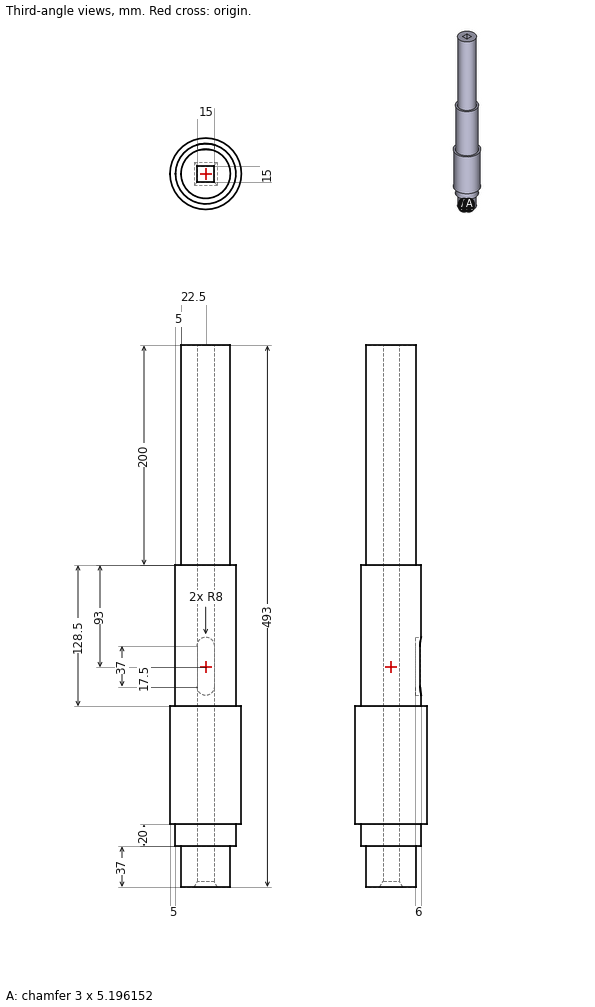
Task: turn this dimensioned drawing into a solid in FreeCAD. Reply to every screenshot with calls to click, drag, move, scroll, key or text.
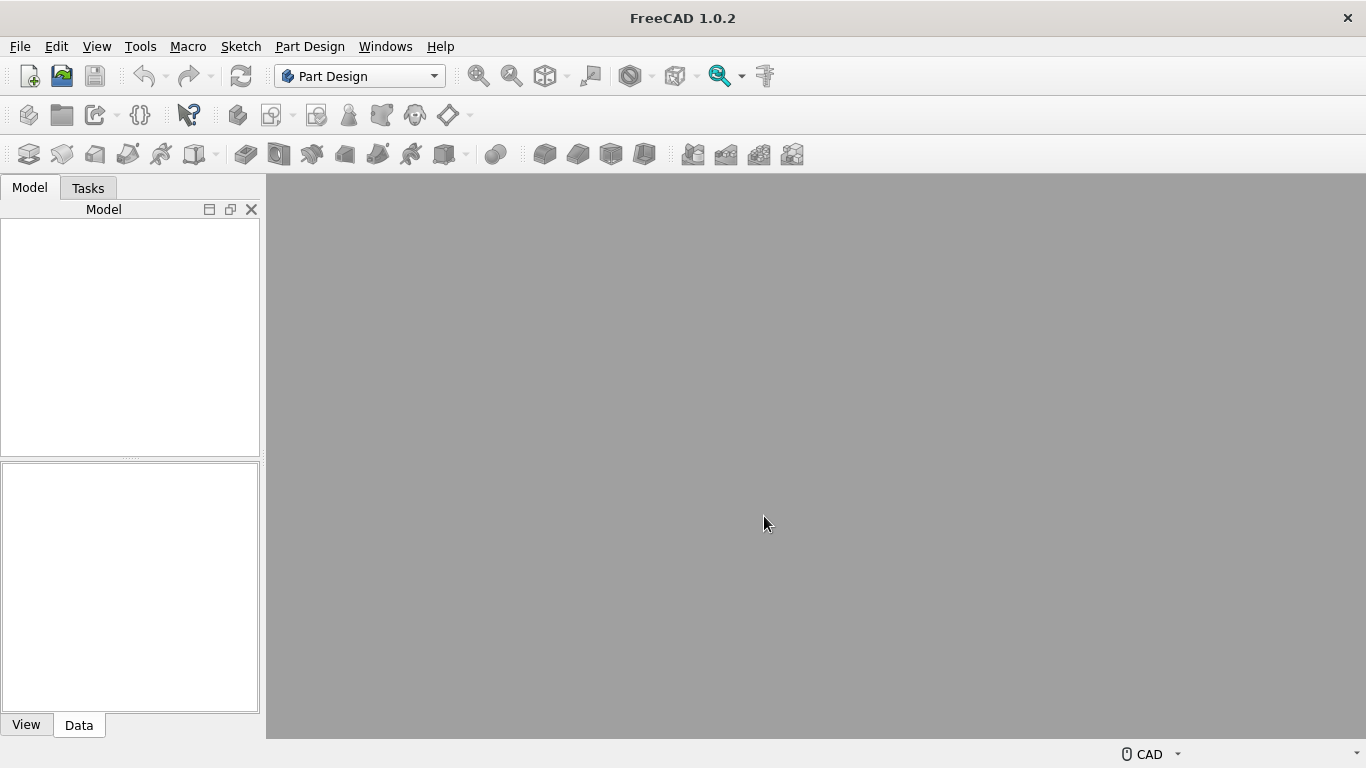
click(29, 76)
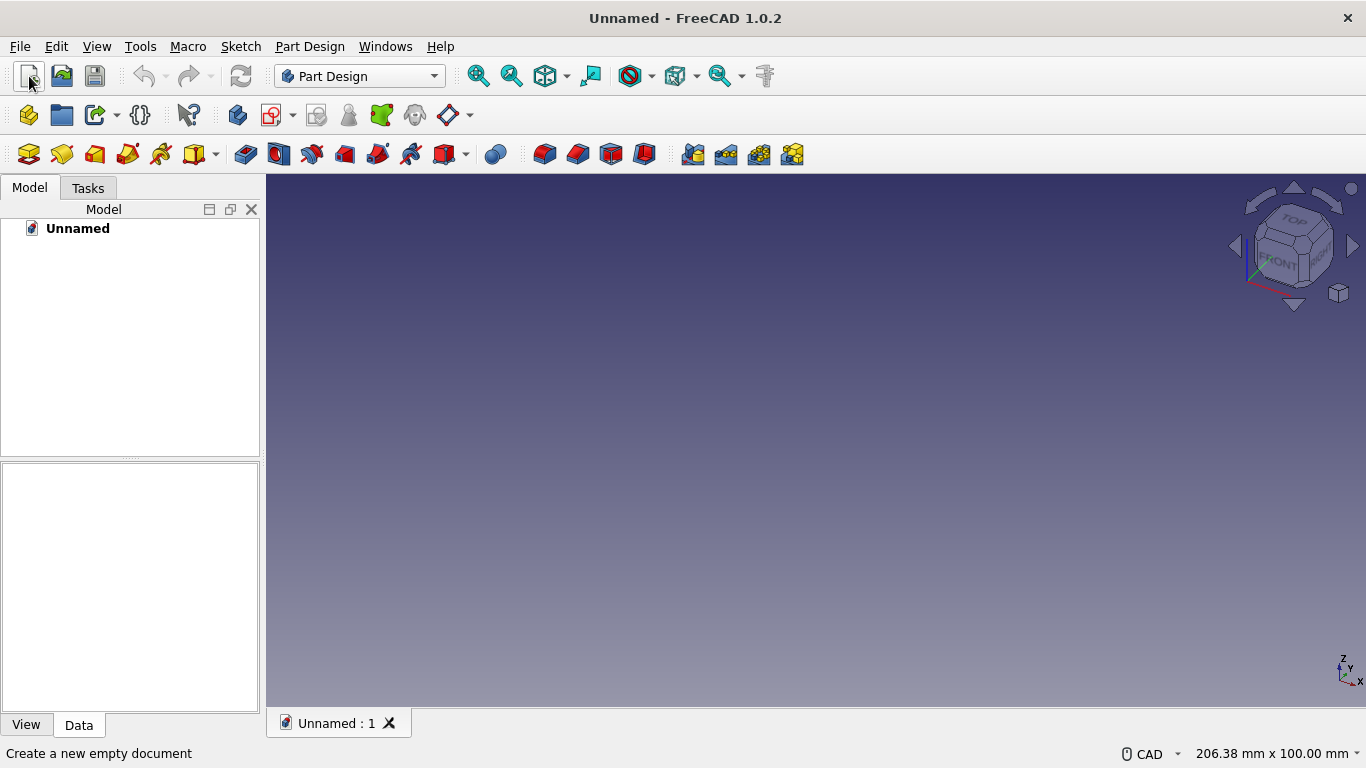
click(270, 116)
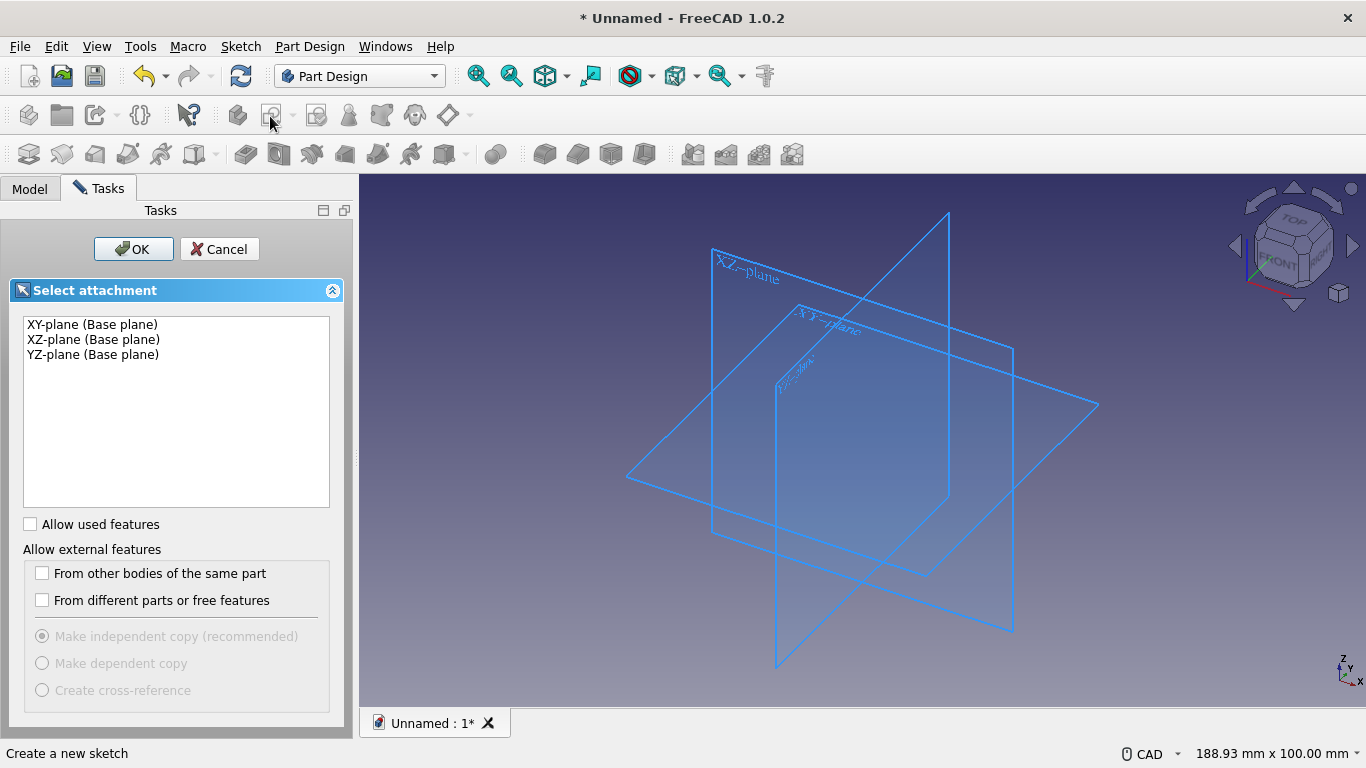
click(84, 340)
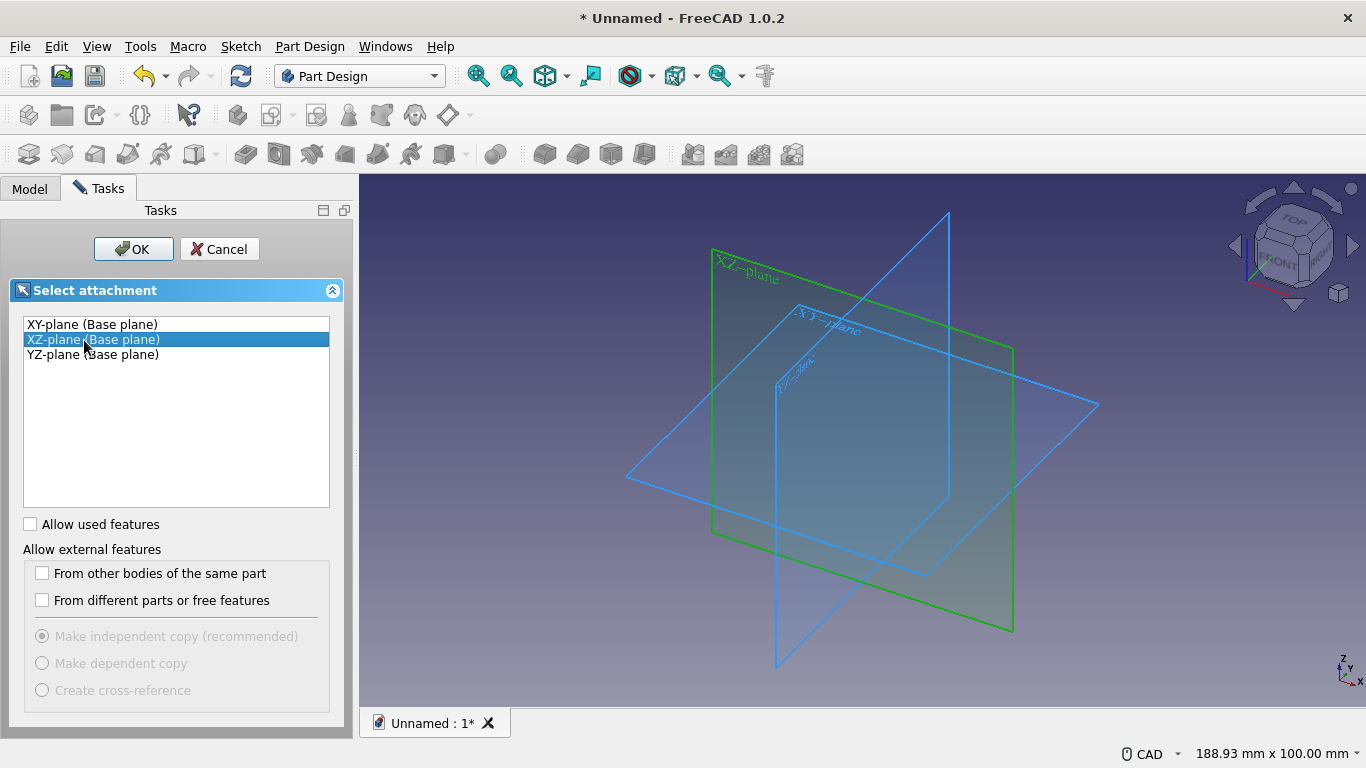
click(134, 249)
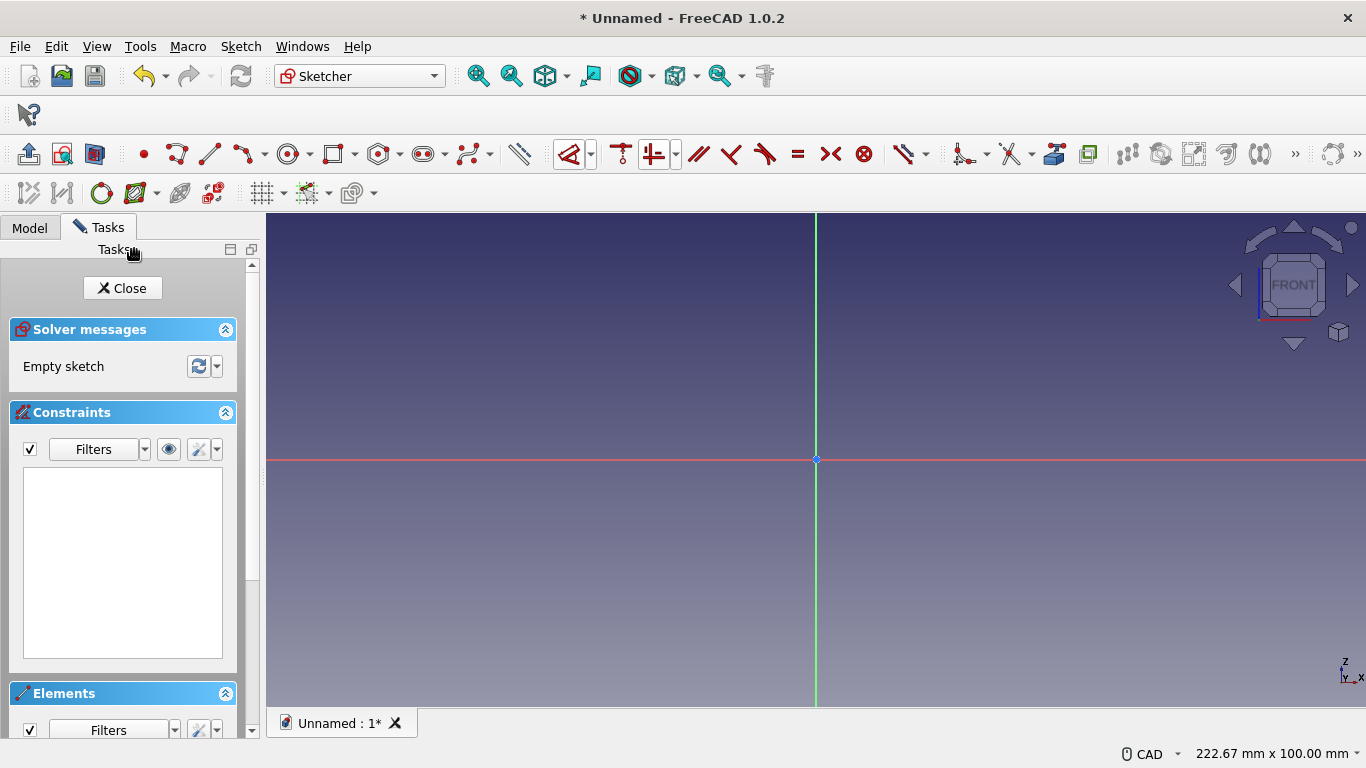
scroll(749, 496, down, 10)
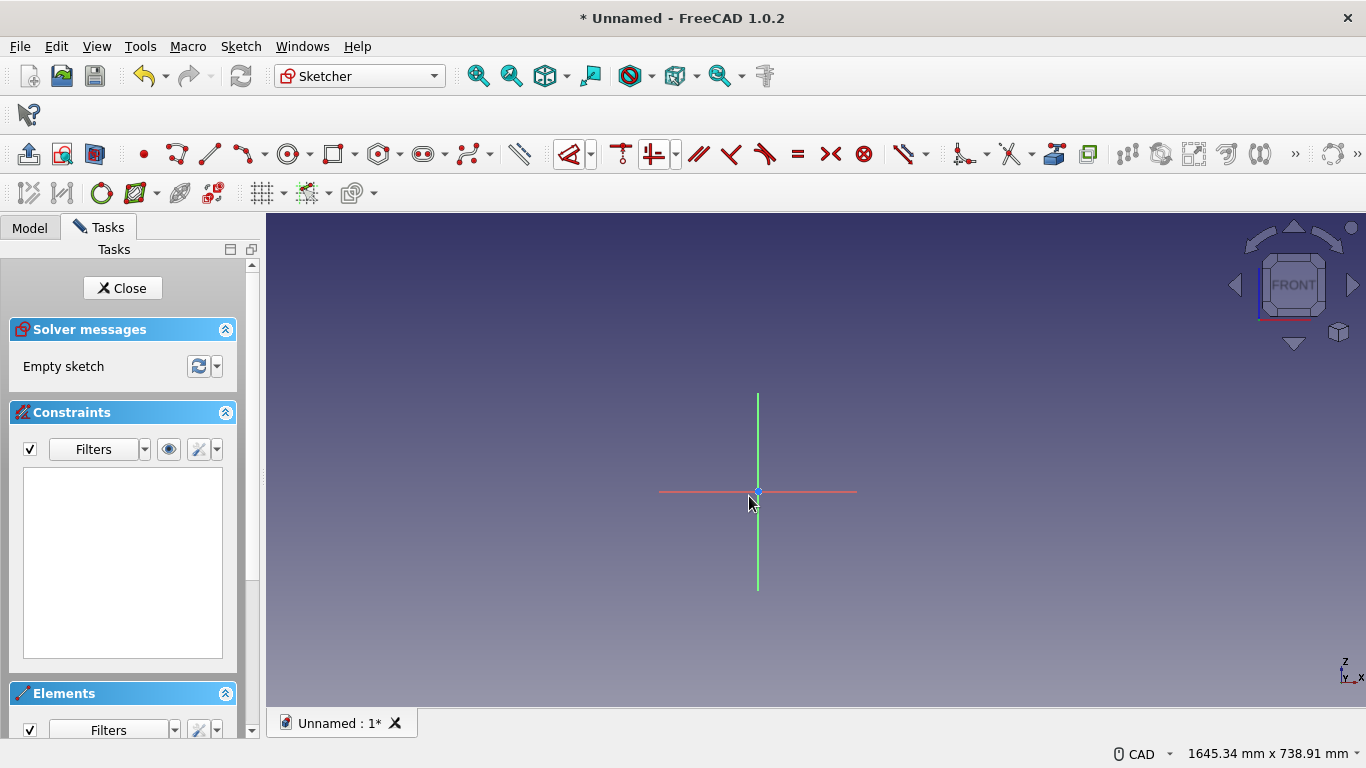
key(g)
key(m)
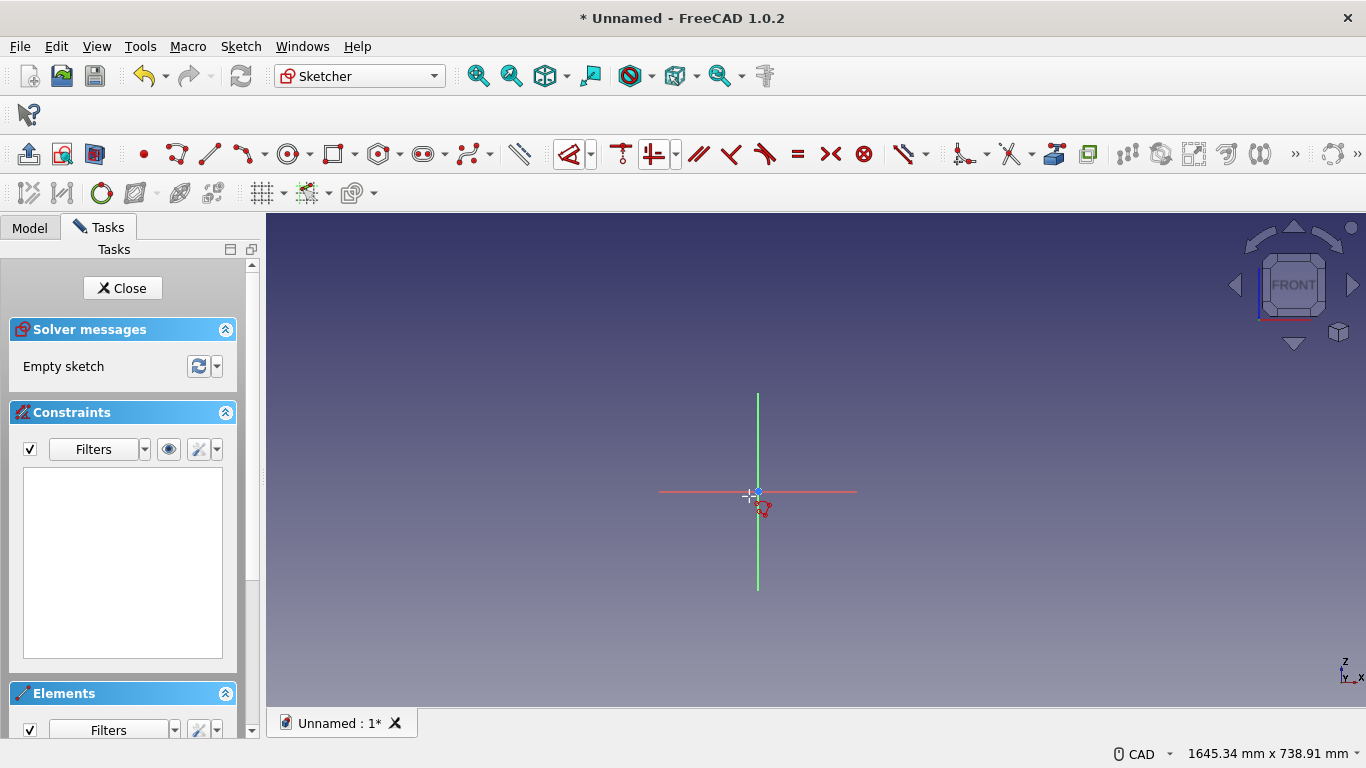
click(740, 515)
click(740, 429)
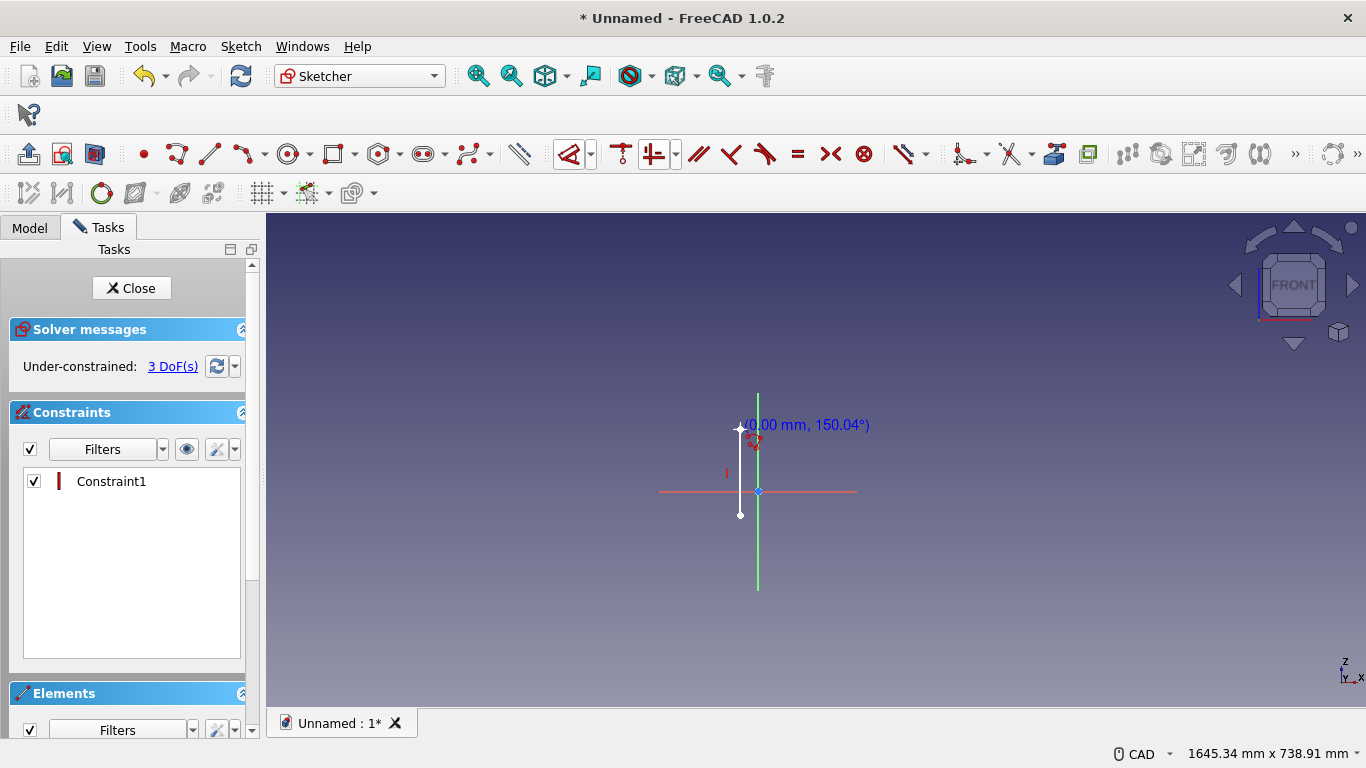
scroll(743, 429, up, 8)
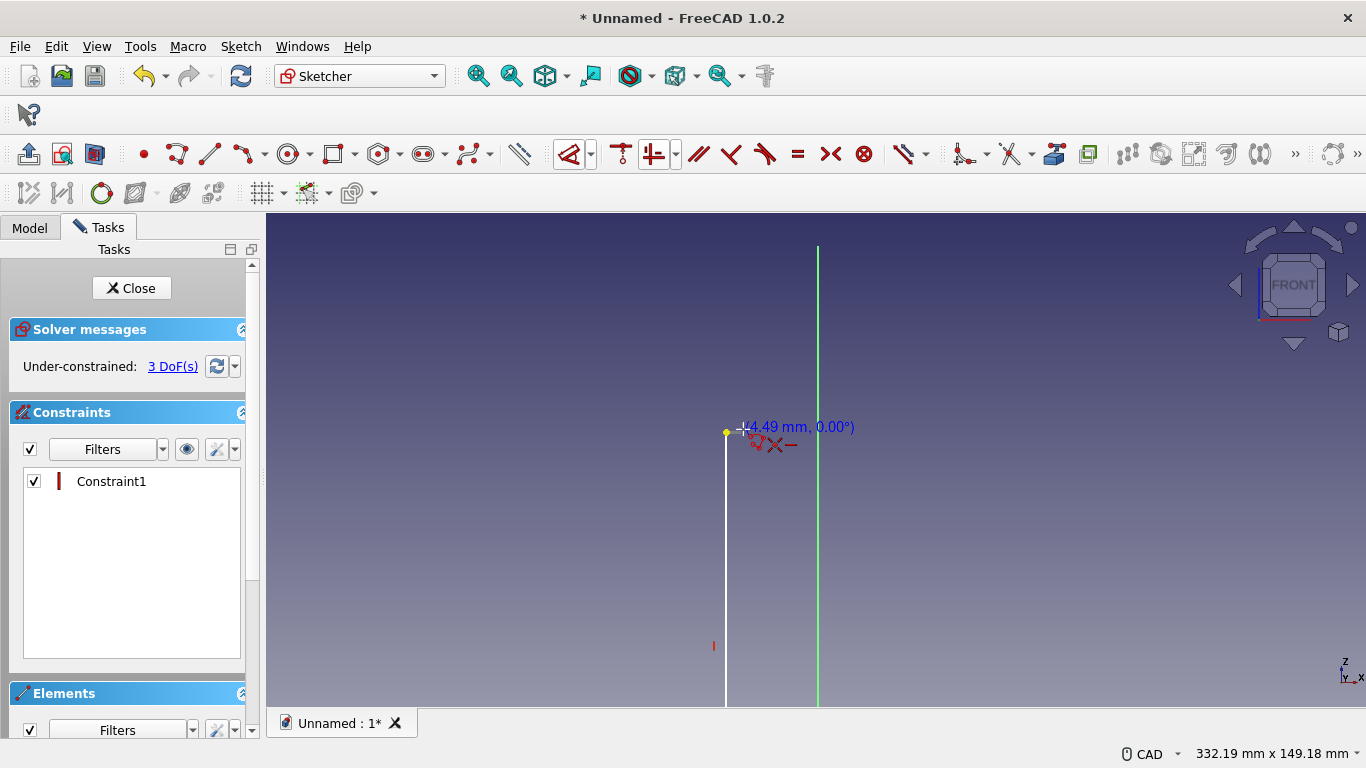
click(743, 427)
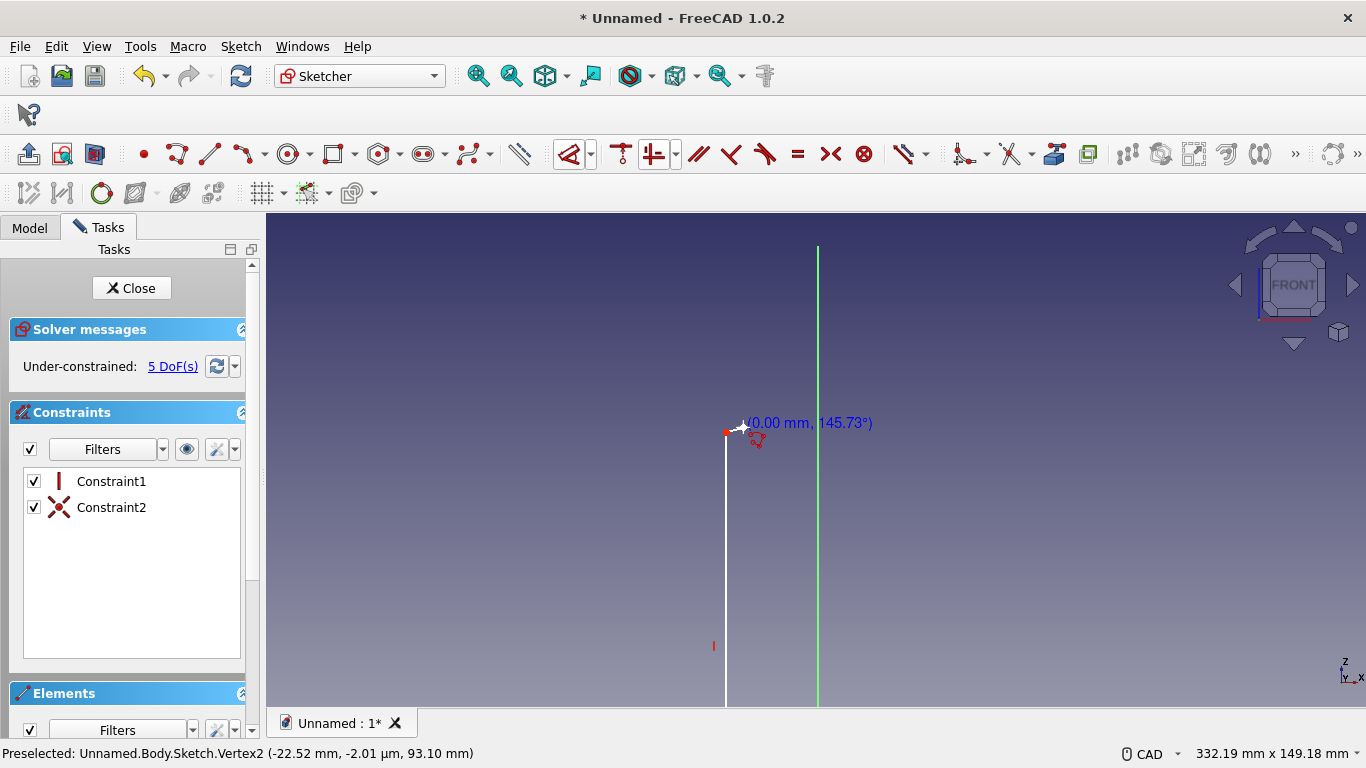
scroll(743, 429, down, 8)